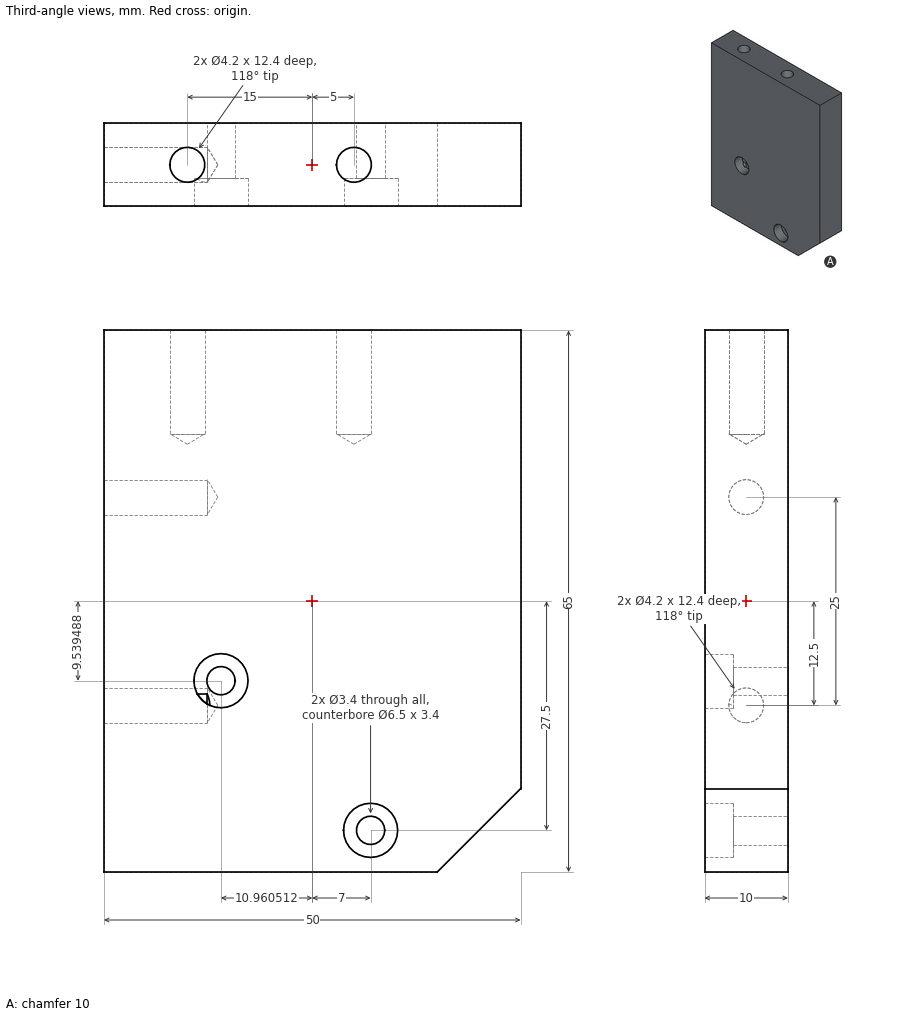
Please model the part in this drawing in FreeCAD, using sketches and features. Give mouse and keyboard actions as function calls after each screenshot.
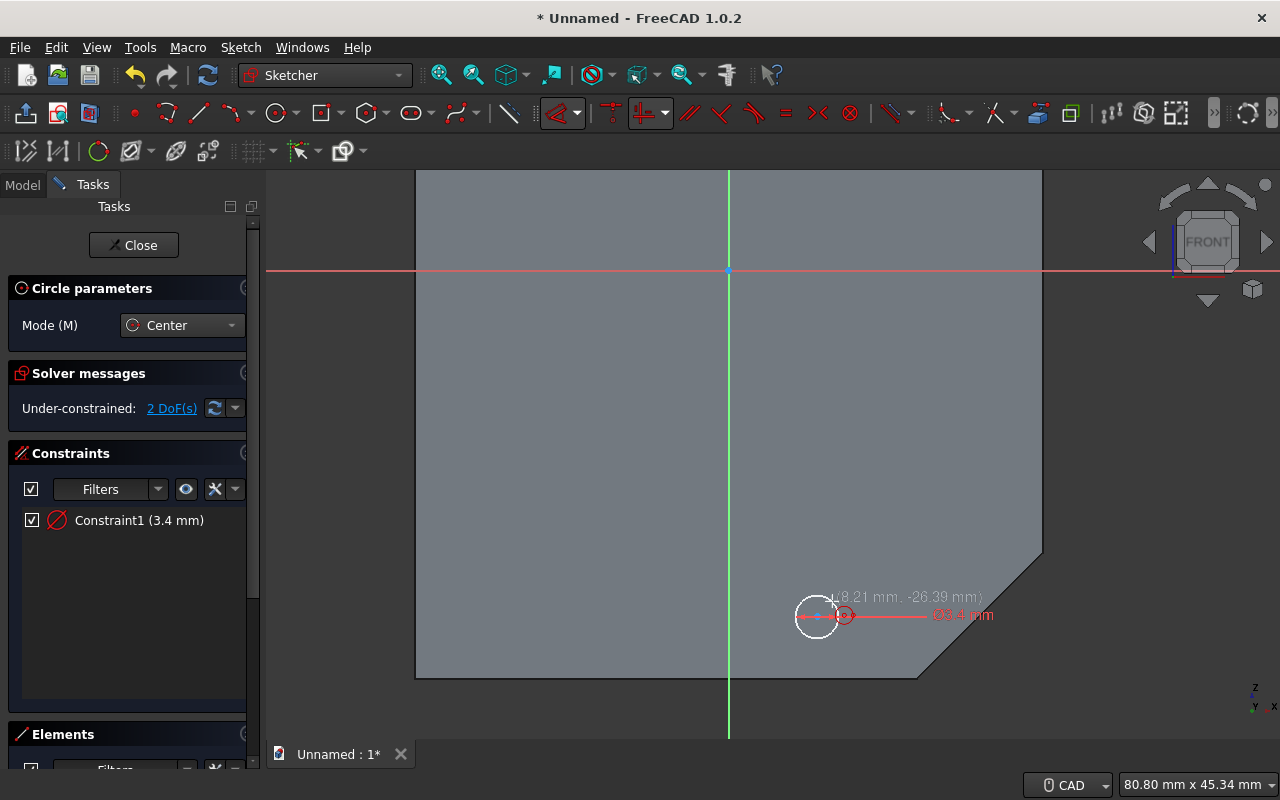
click(591, 391)
move(607, 375)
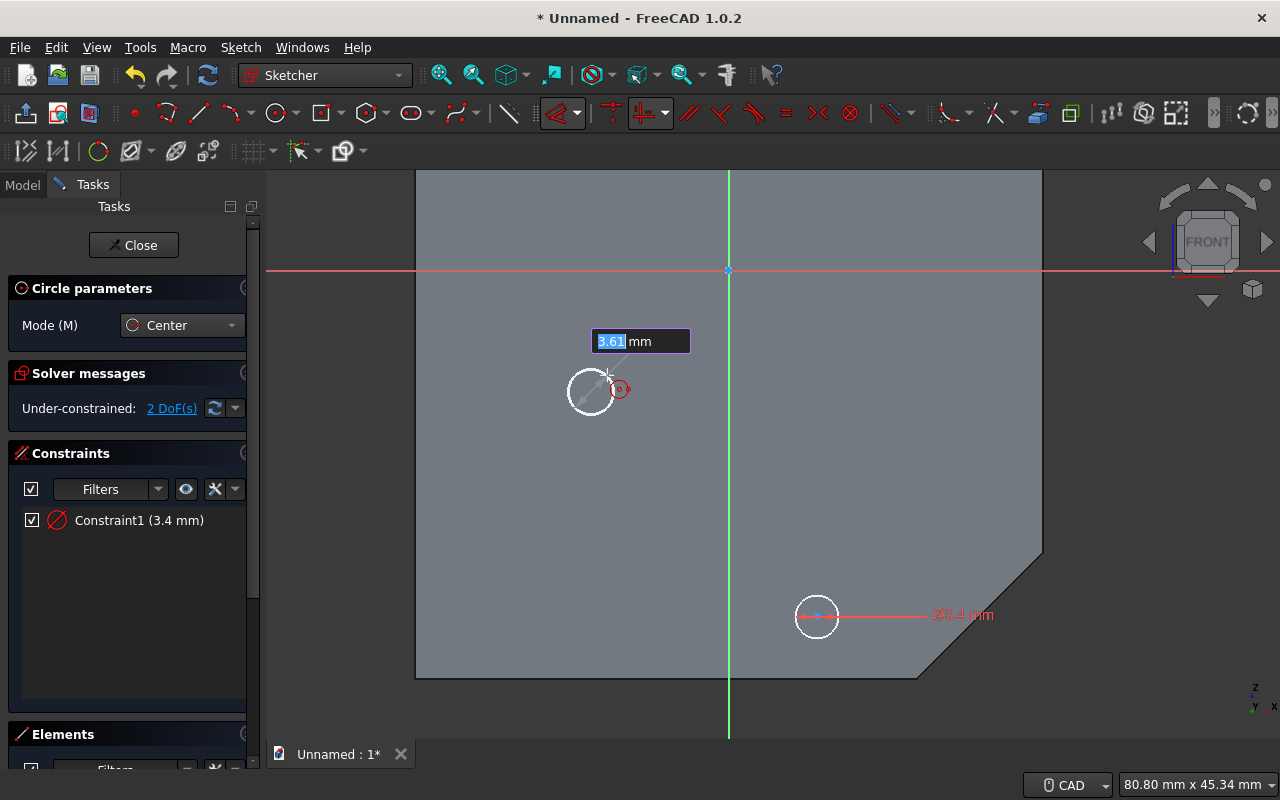
text(3.4)
key(Return)
key(Escape)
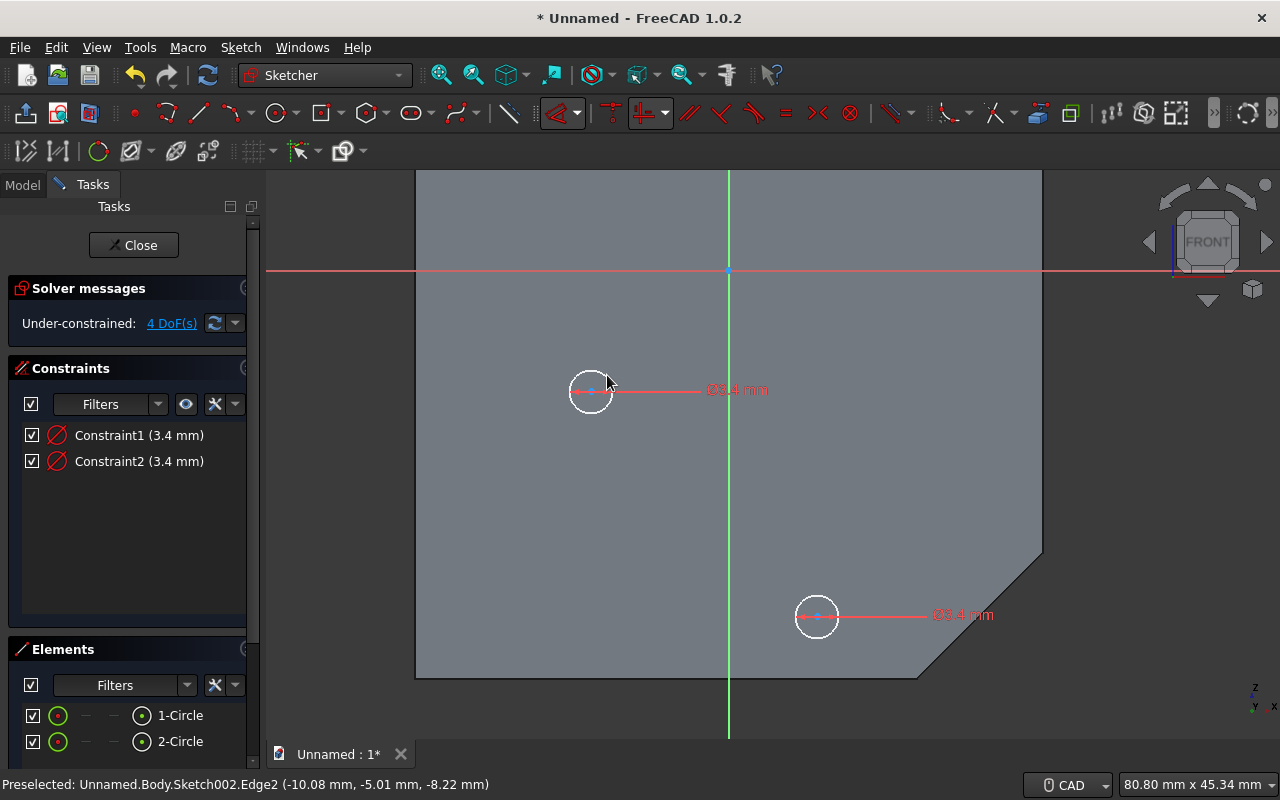
key(d)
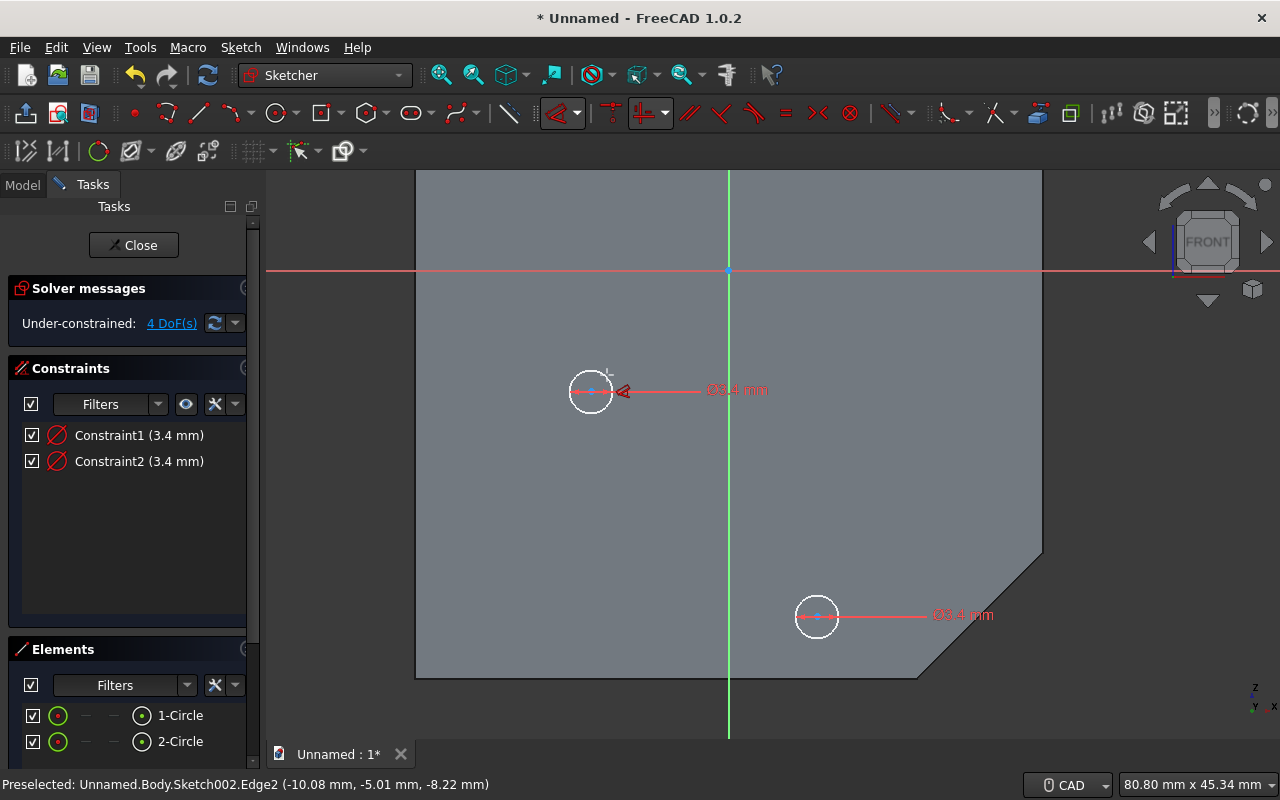
click(817, 617)
click(773, 237)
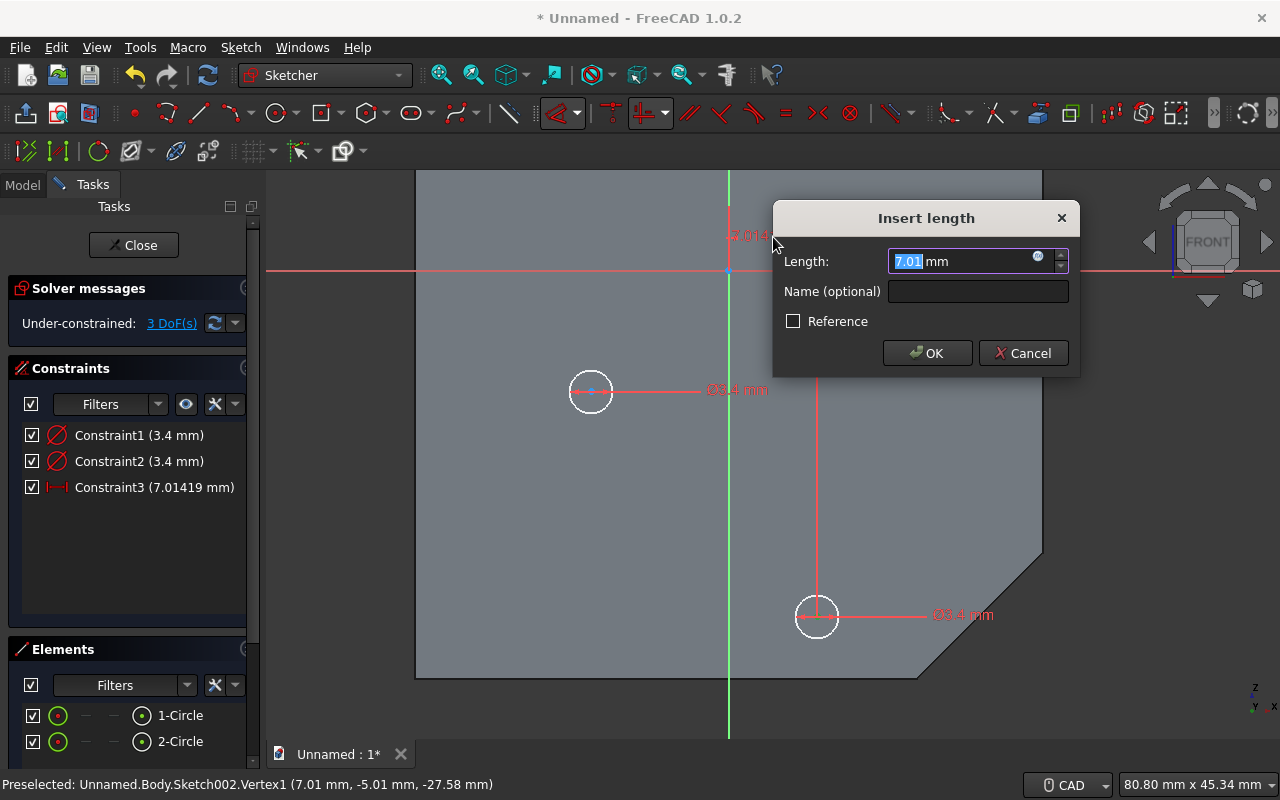
text(7)
key(Return)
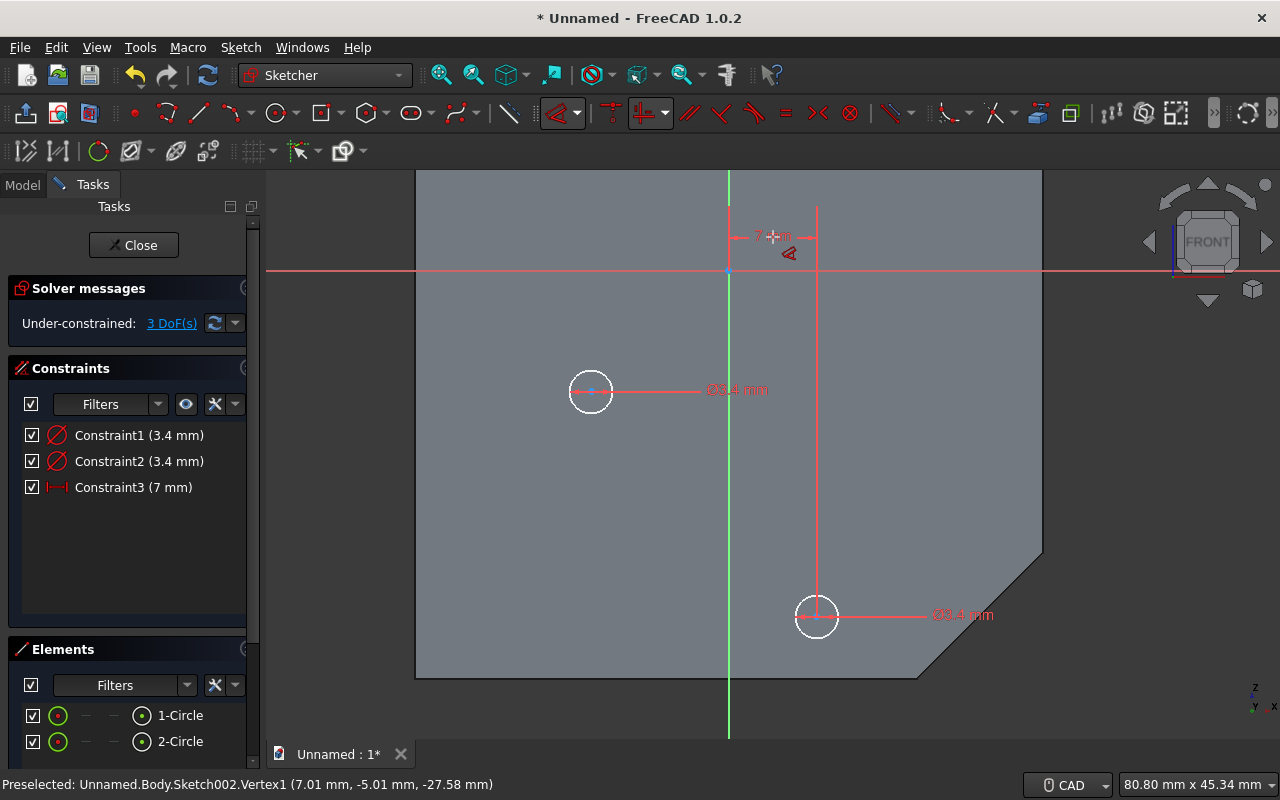
click(817, 617)
click(851, 444)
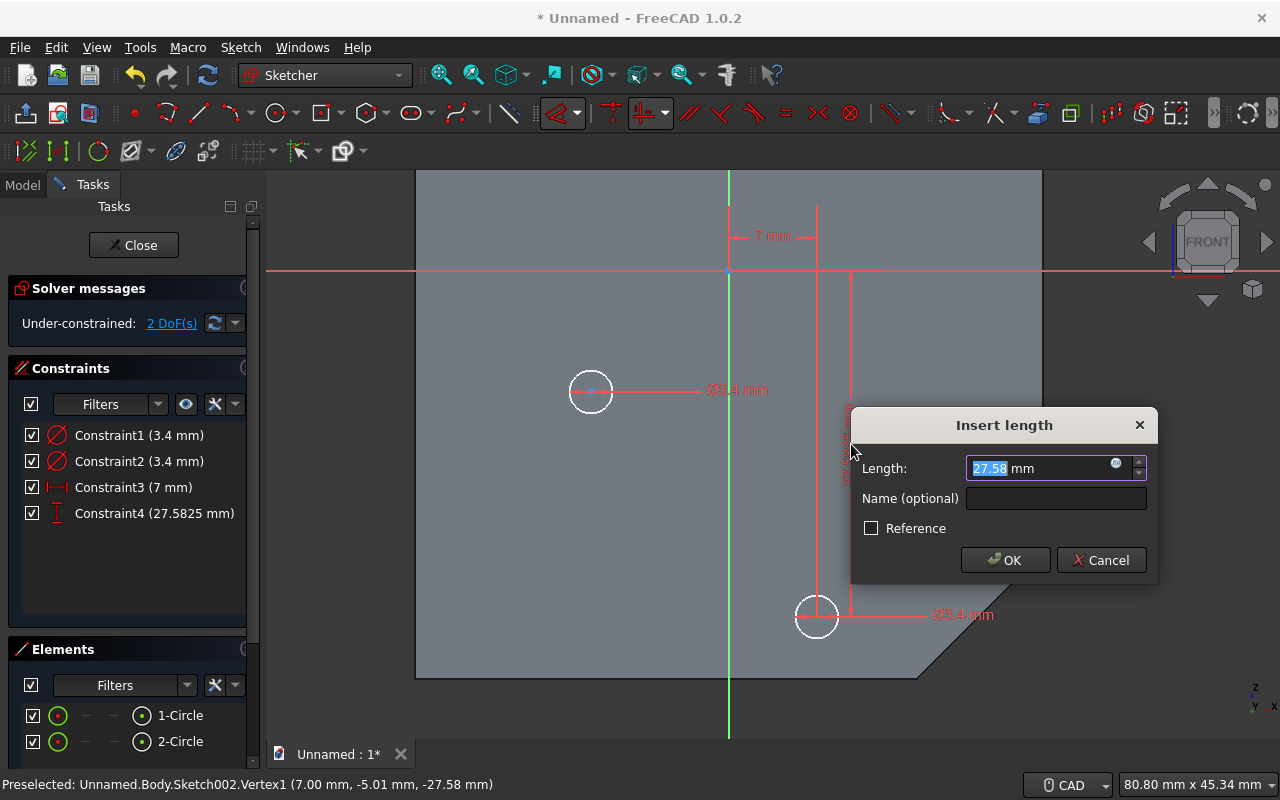
text(27.5)
key(Return)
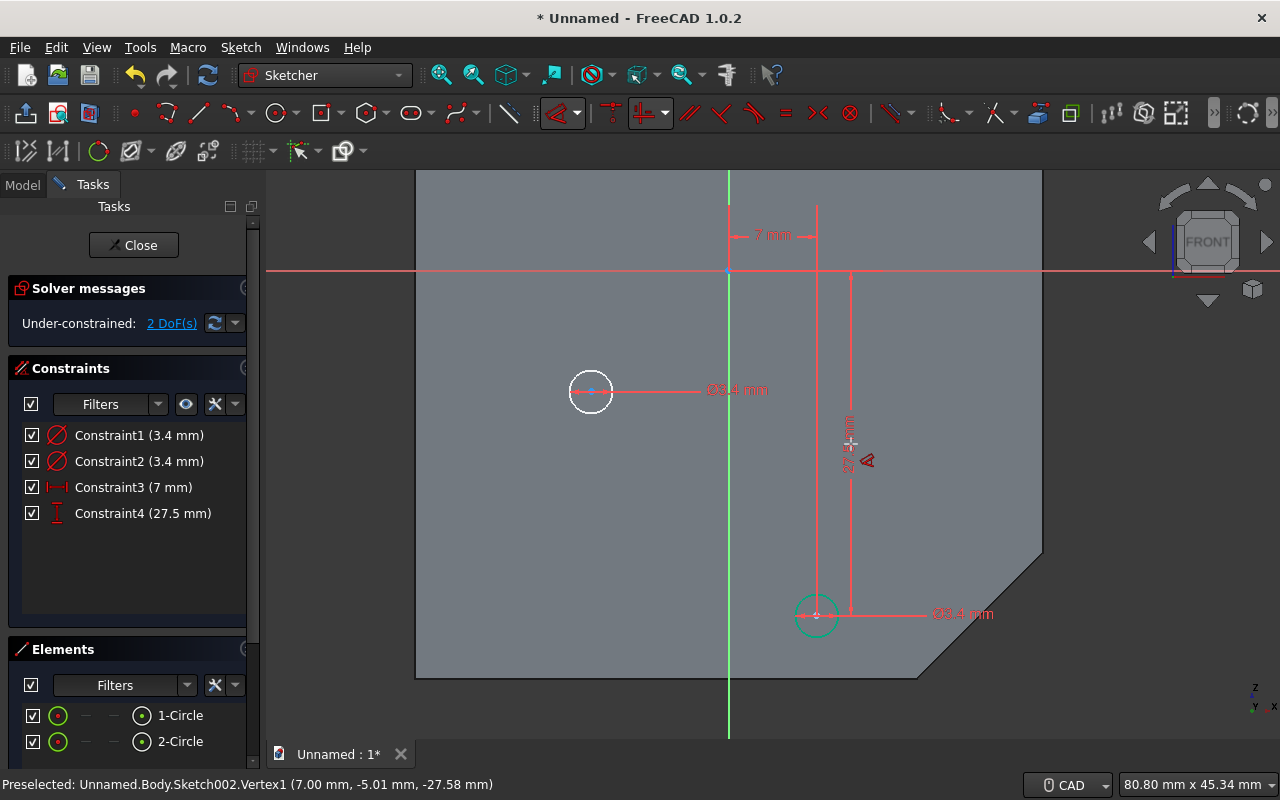
click(591, 392)
click(557, 331)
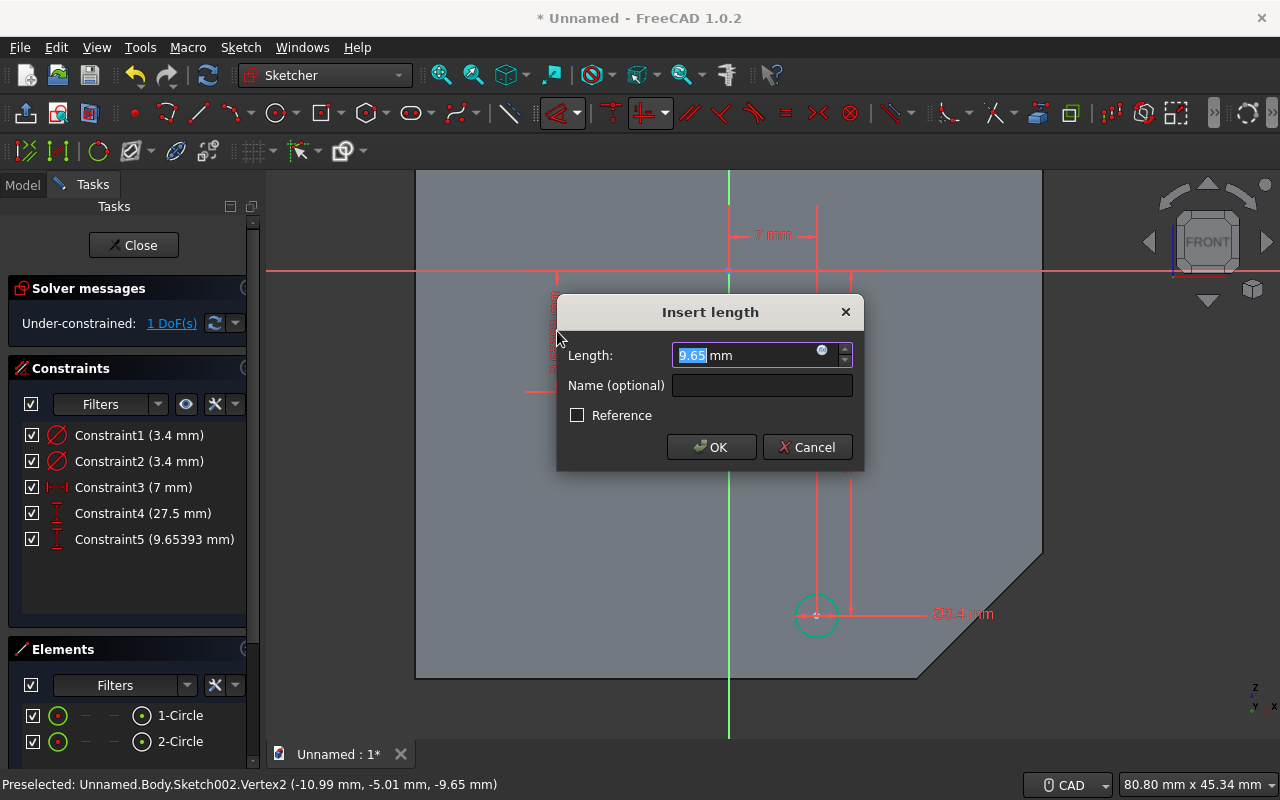
text(9.539488)
key(Return)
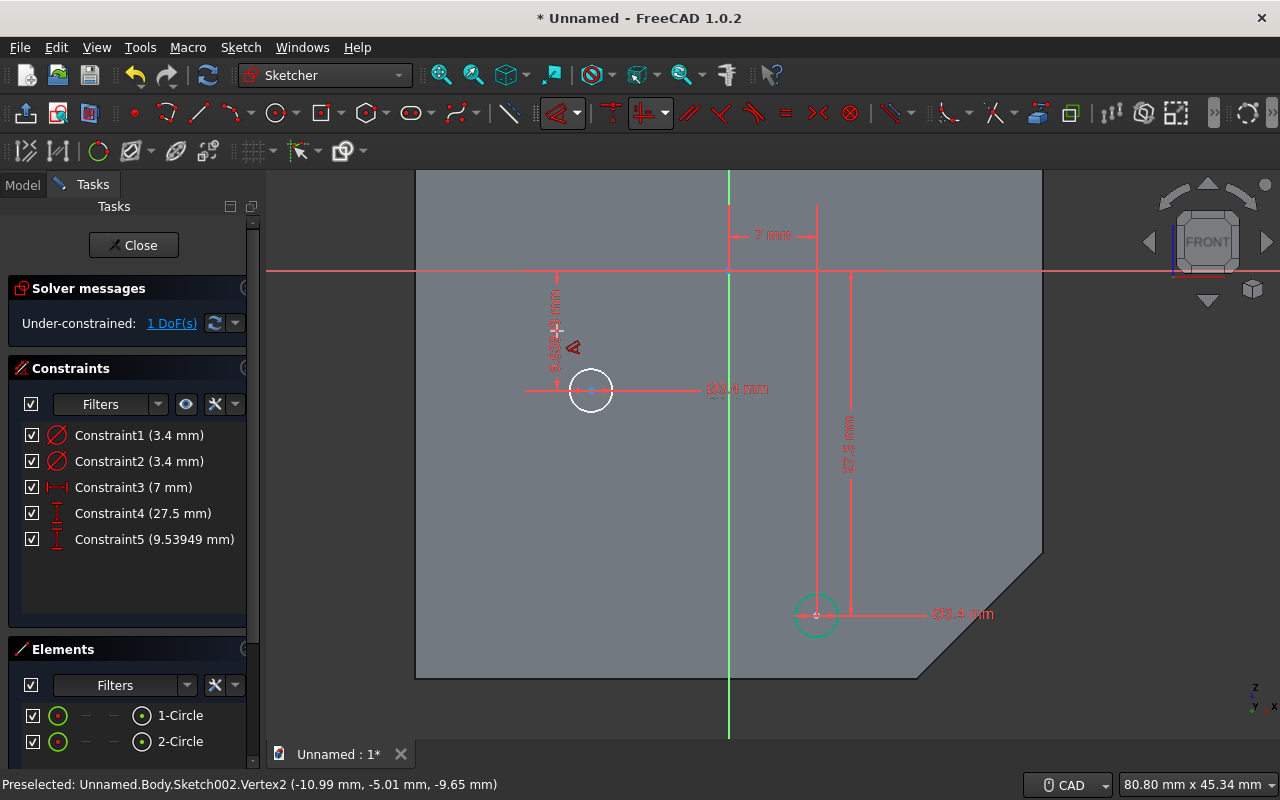
click(591, 391)
click(660, 237)